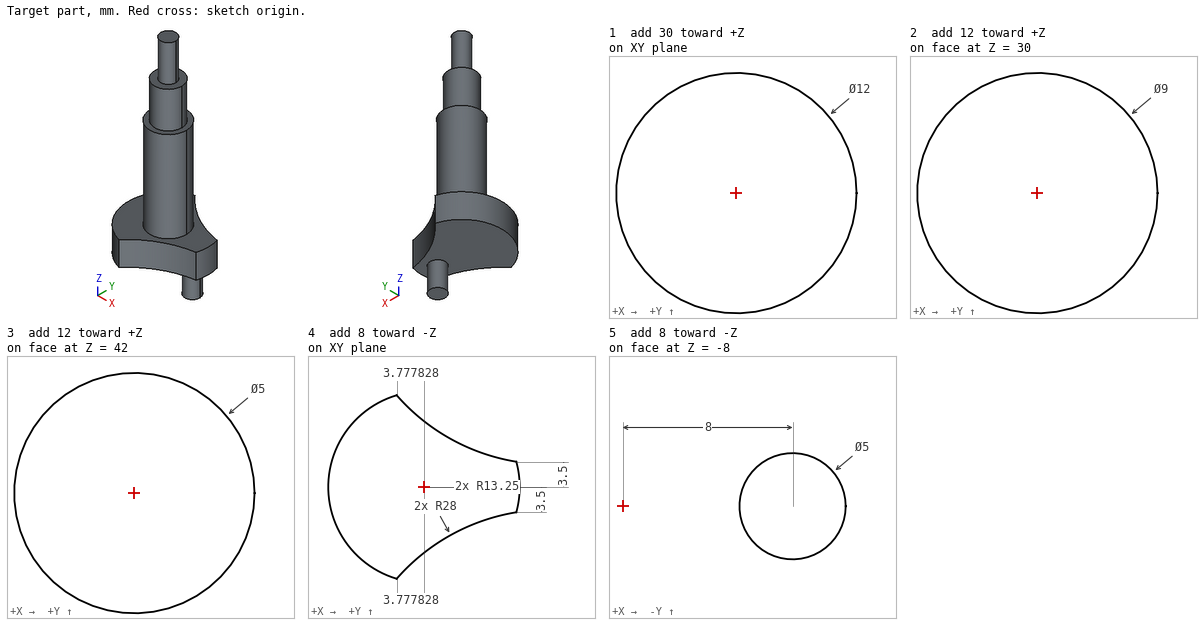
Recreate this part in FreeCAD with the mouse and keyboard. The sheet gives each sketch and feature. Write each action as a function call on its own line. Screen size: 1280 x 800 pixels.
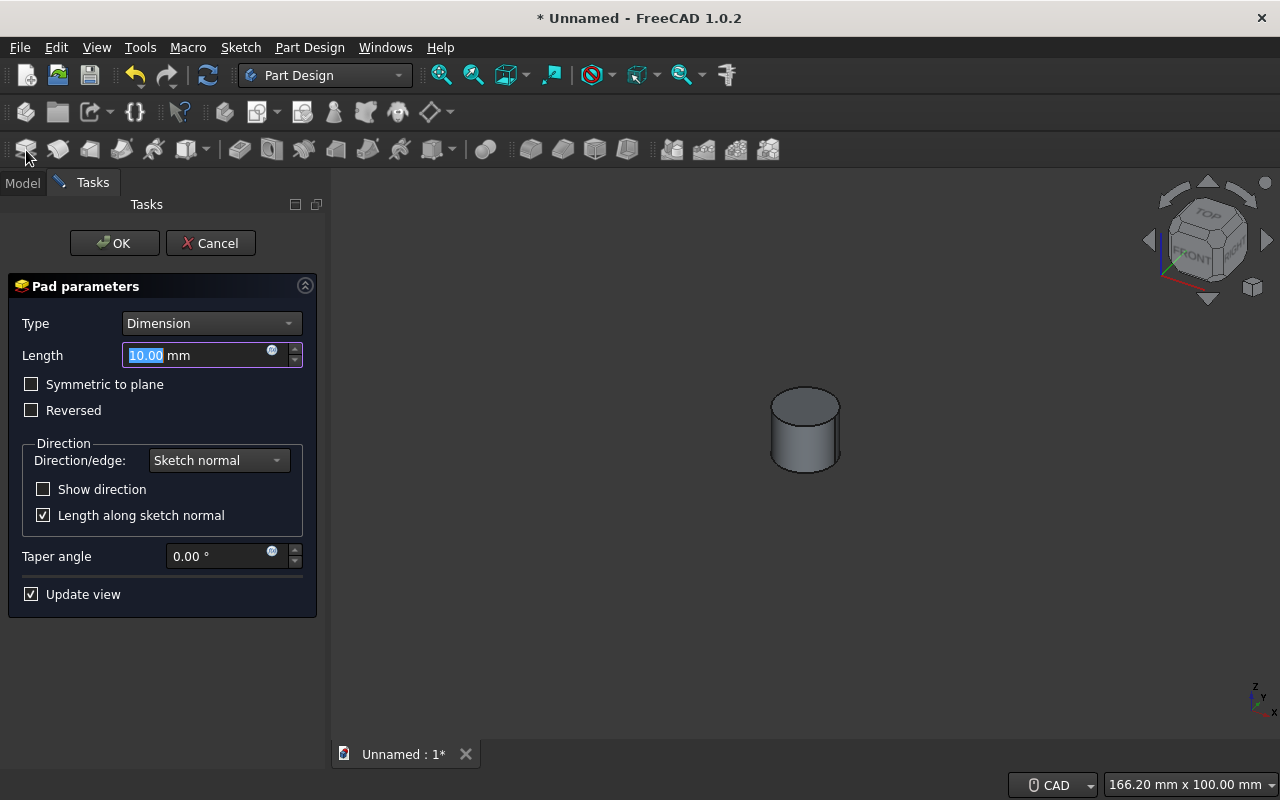
text(30)
key(Tab)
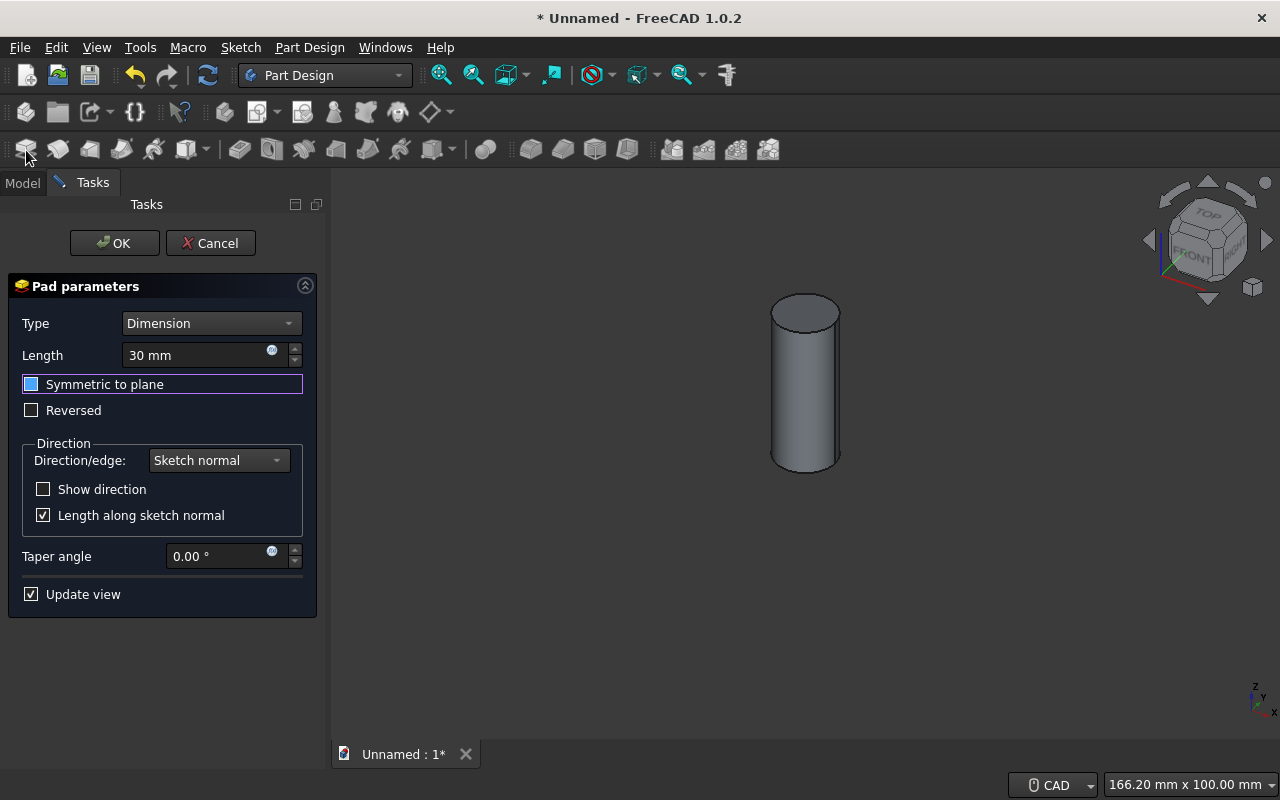
click(115, 243)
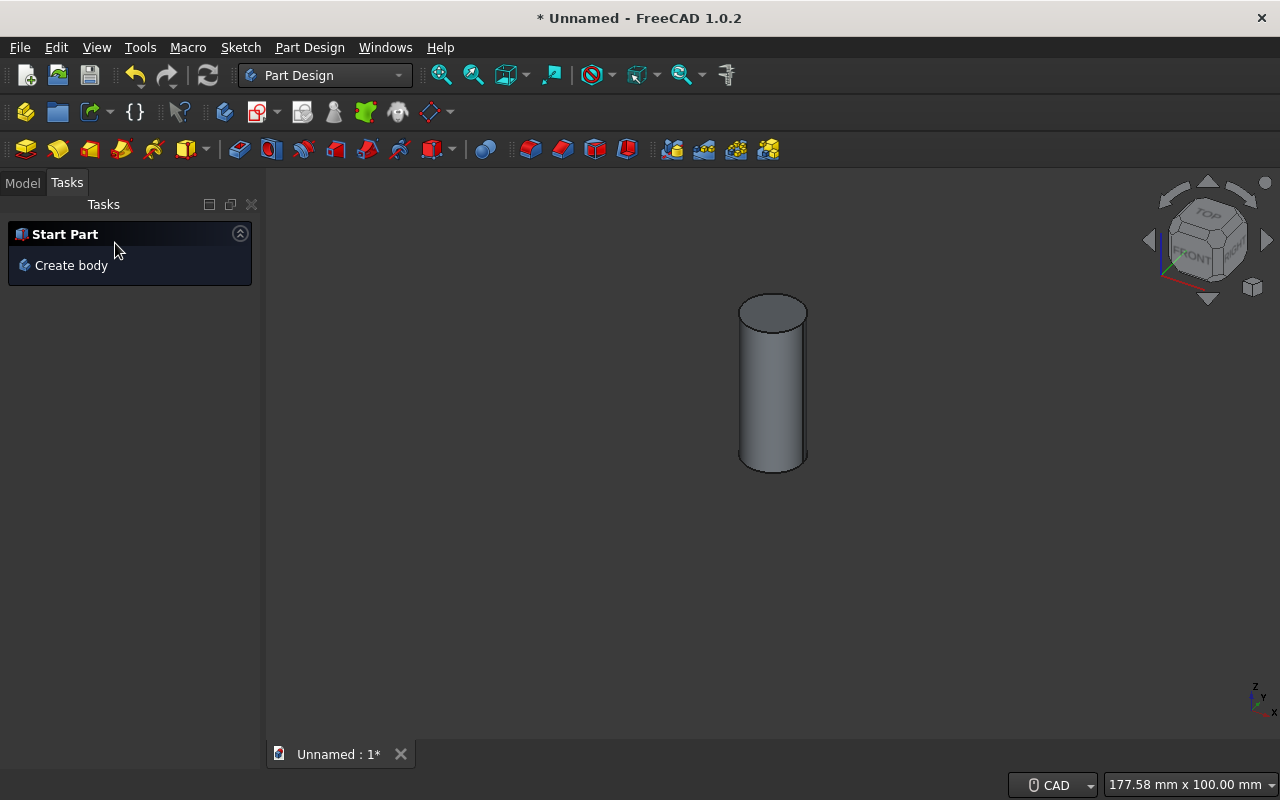
click(442, 76)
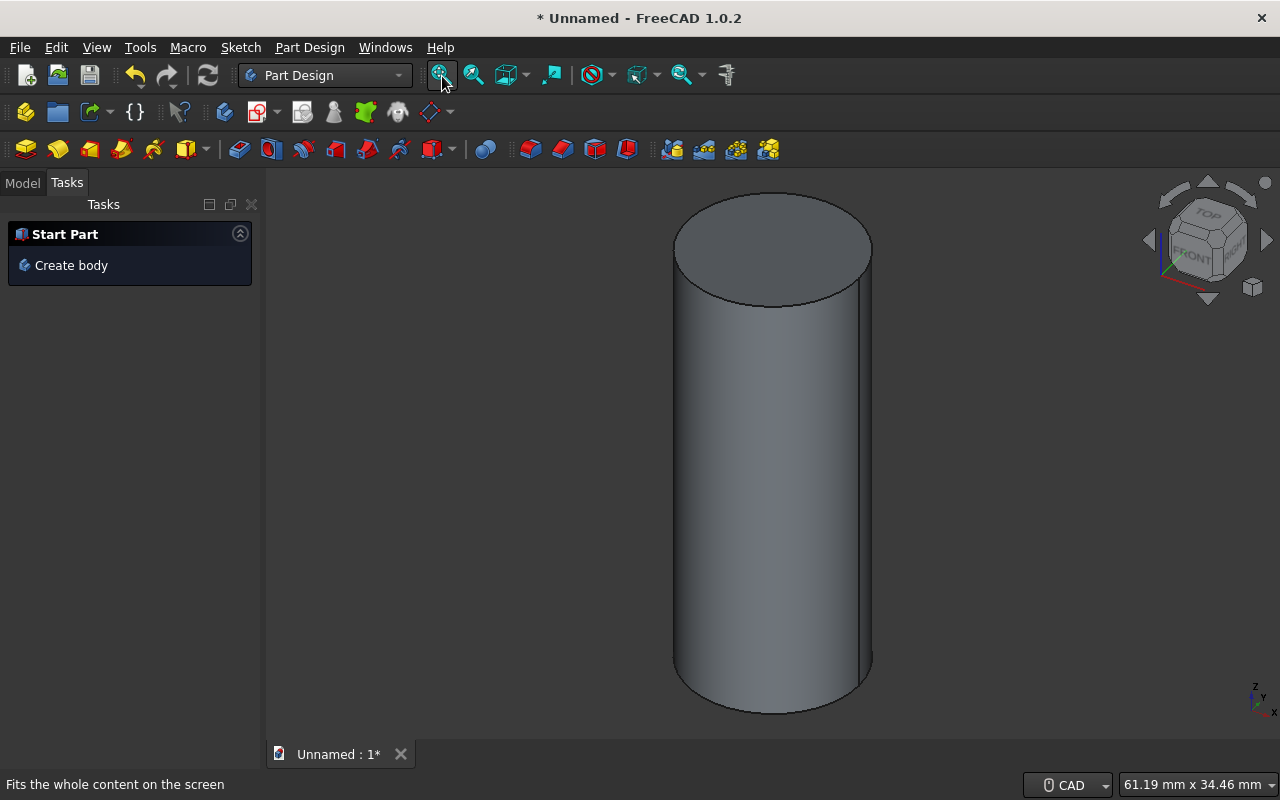
click(773, 249)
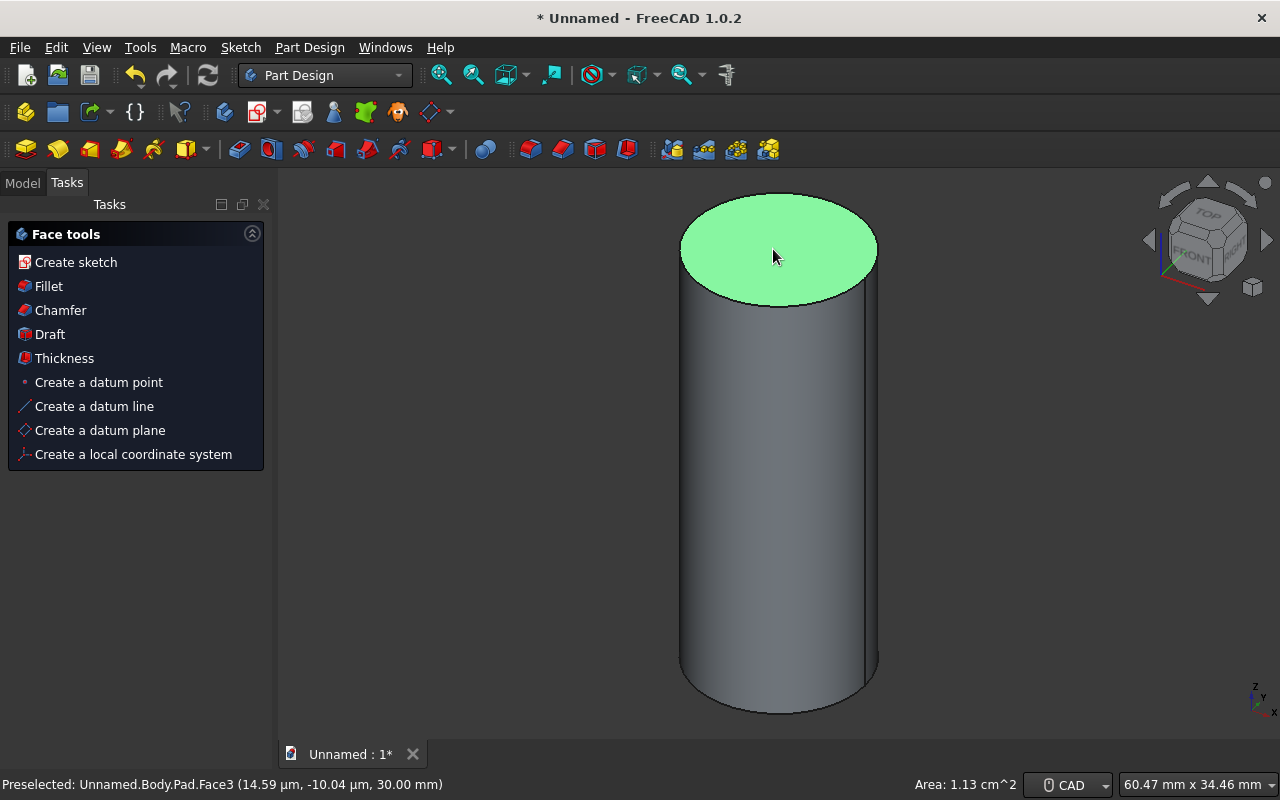
click(258, 112)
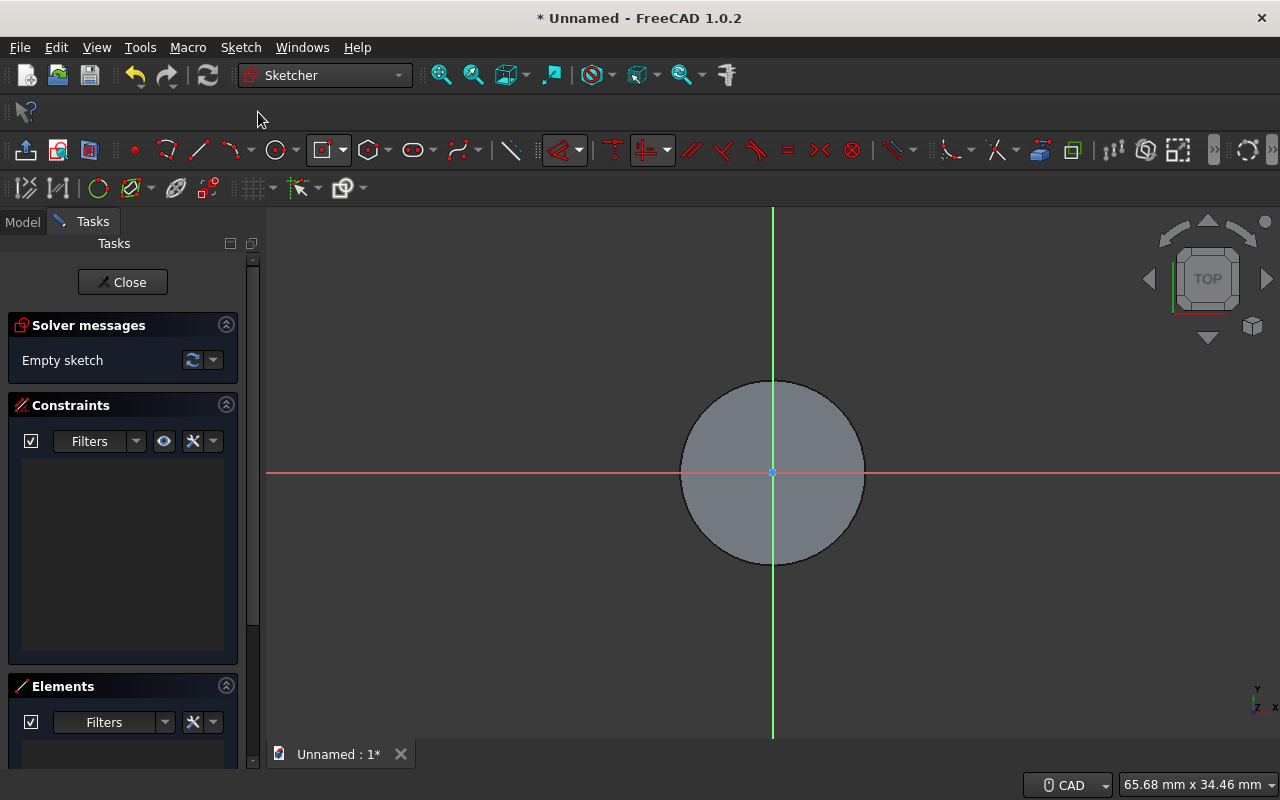
scroll(829, 473, up, 4)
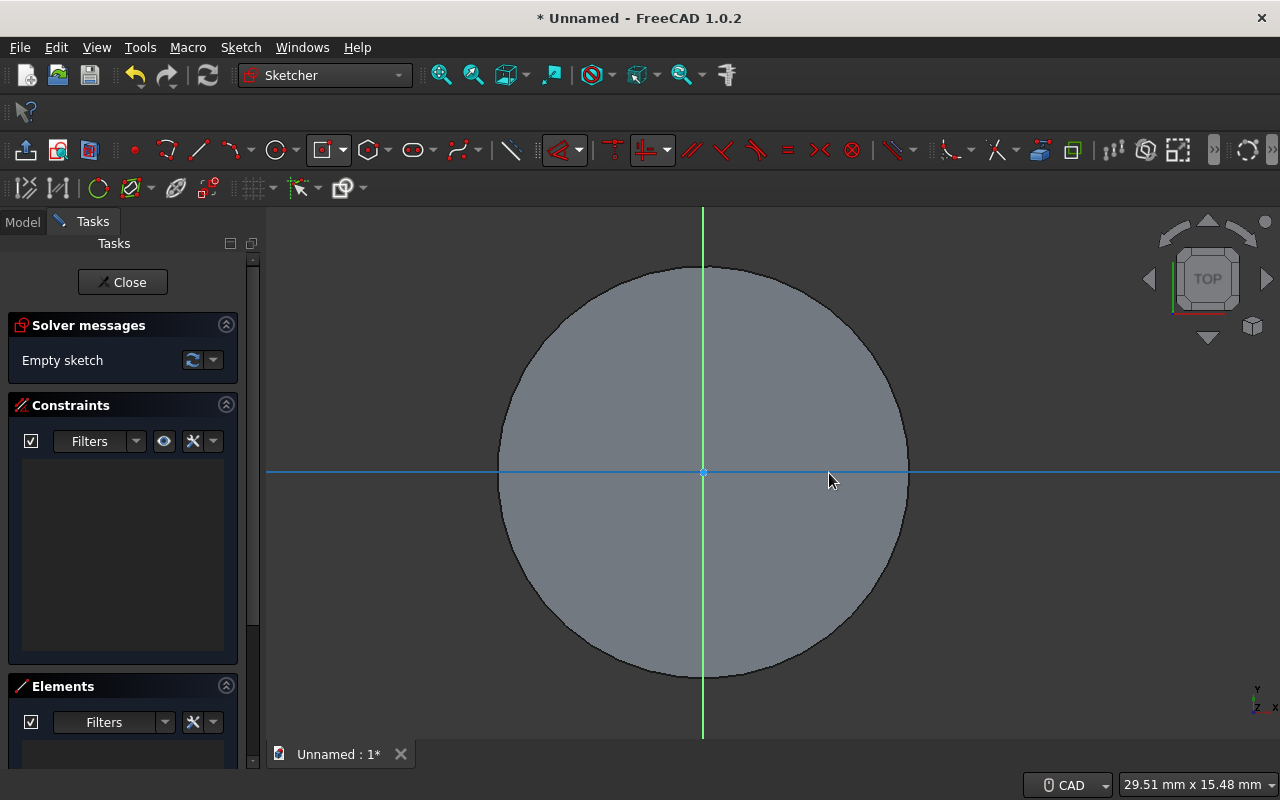
click(276, 150)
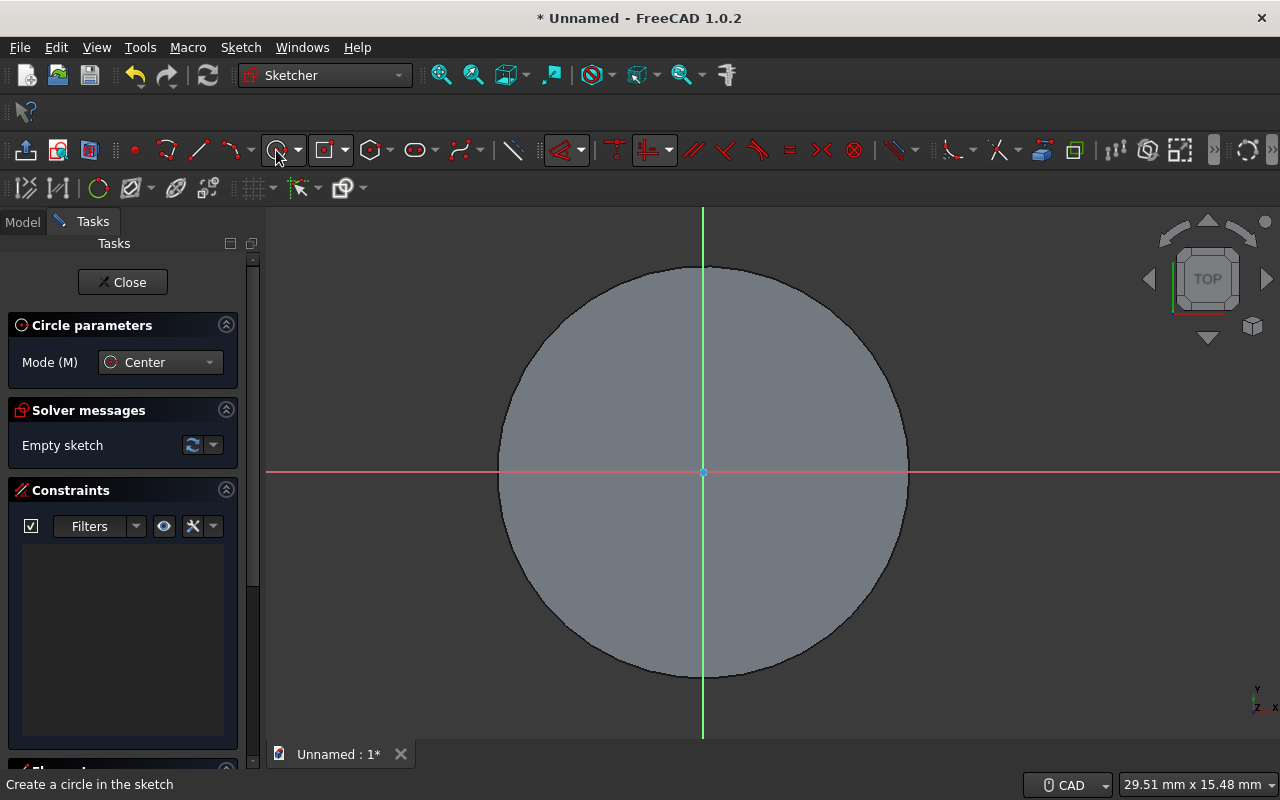
click(703, 472)
move(813, 363)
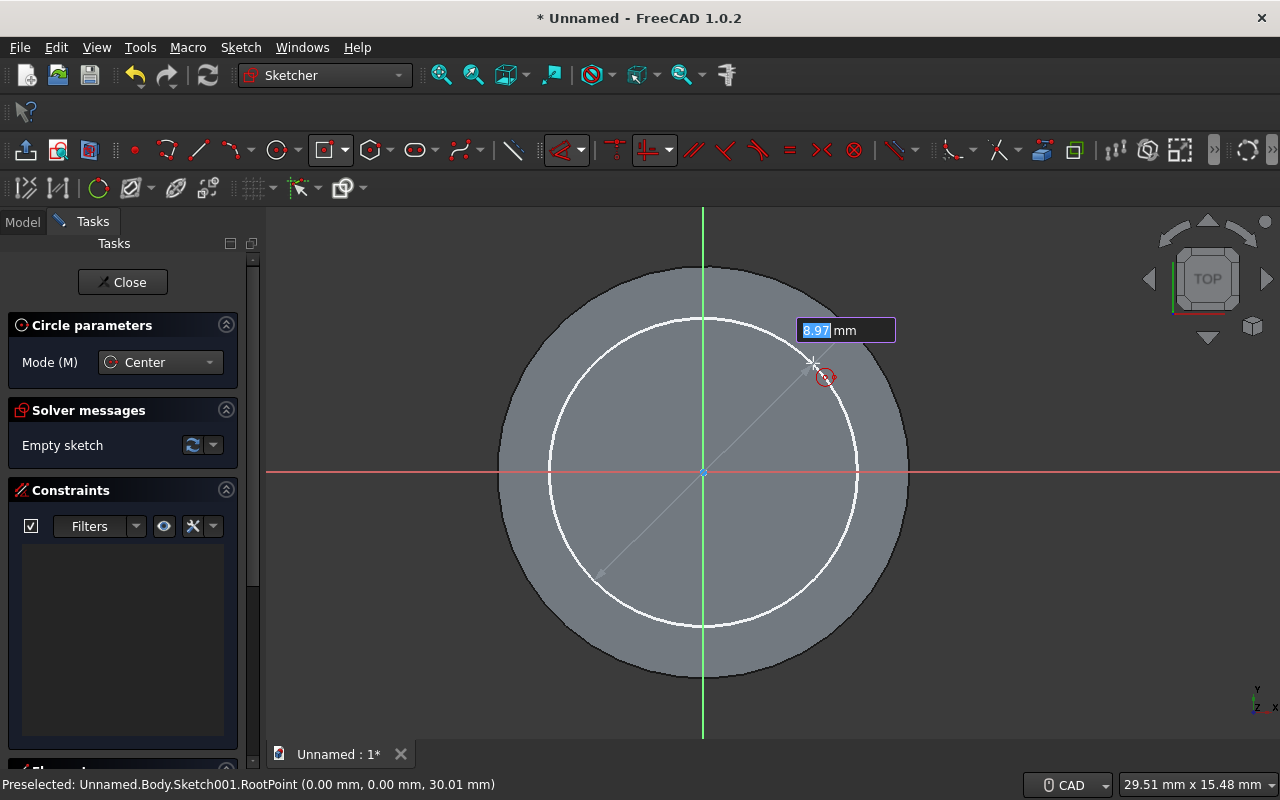
text(9)
key(Return)
key(Escape)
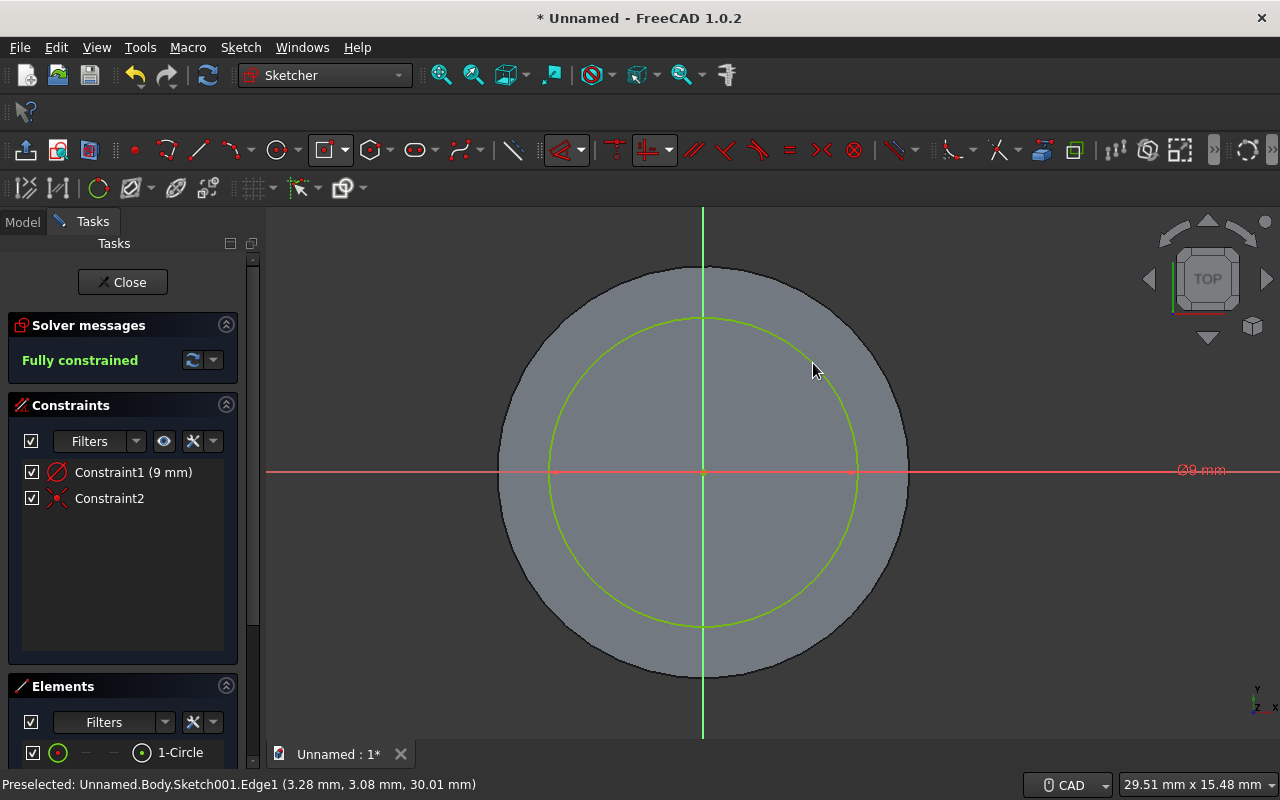
click(123, 282)